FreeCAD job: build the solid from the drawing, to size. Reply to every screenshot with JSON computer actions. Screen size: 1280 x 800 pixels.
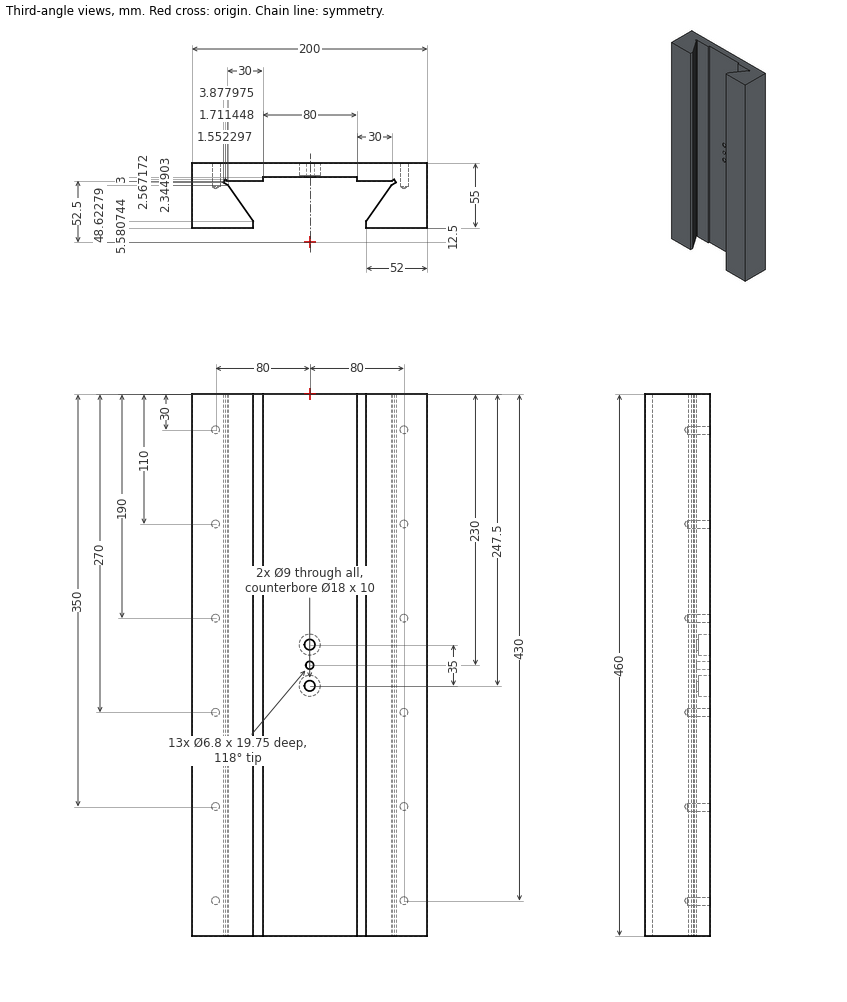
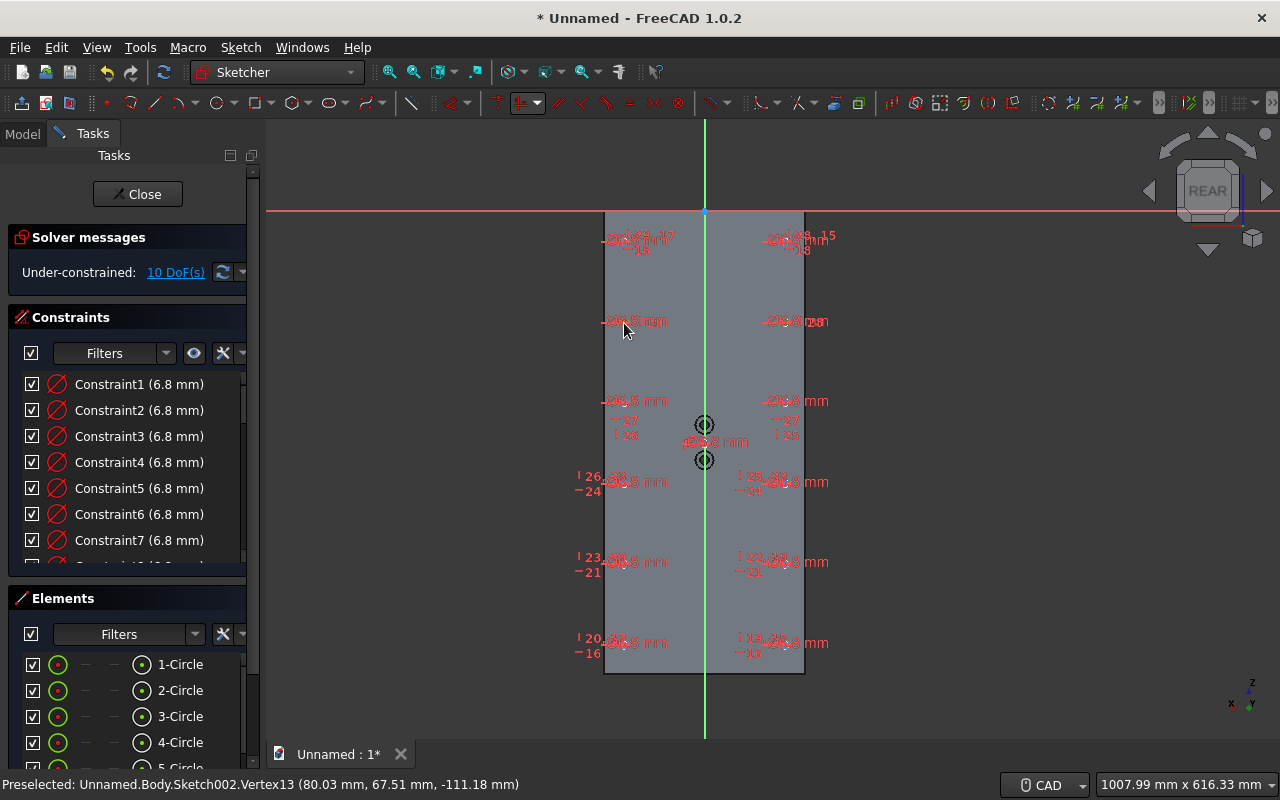
{"action": "key", "text": "h"}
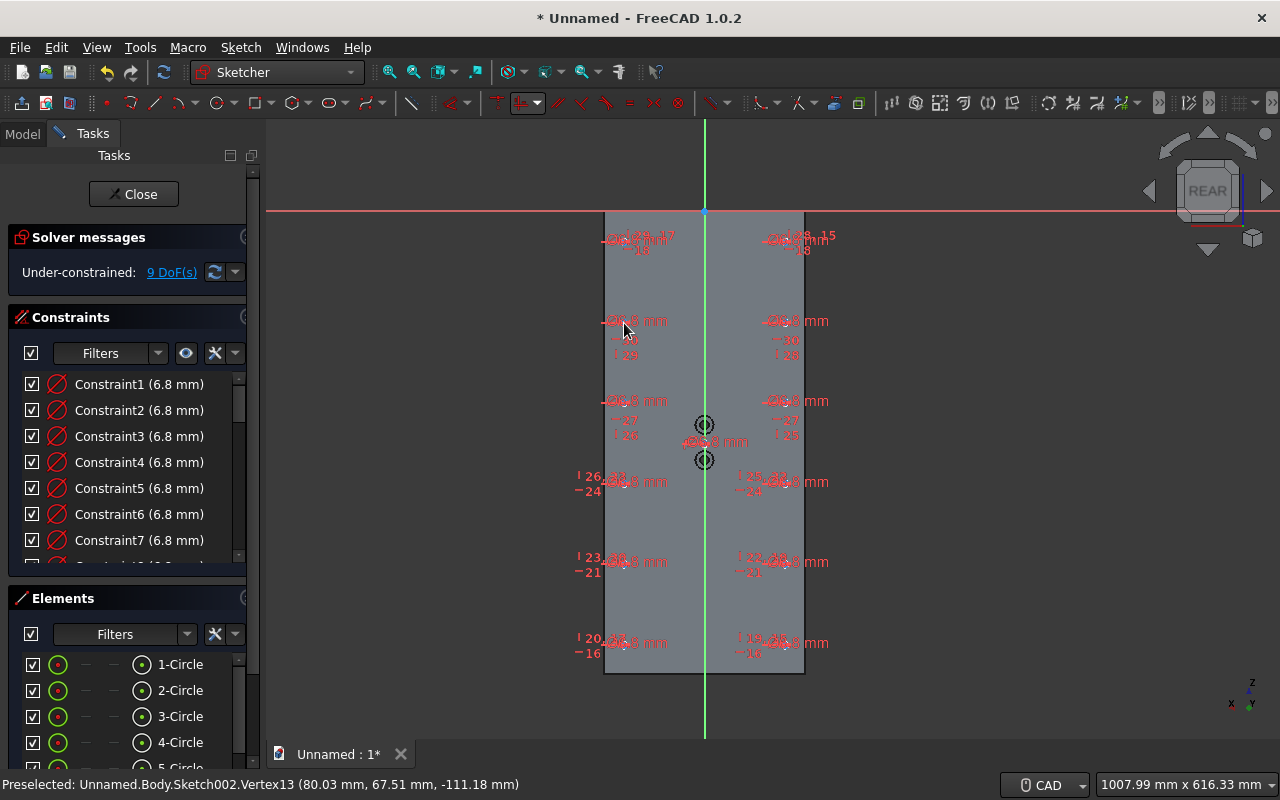
{"action": "left_click", "coordinate": [450, 104]}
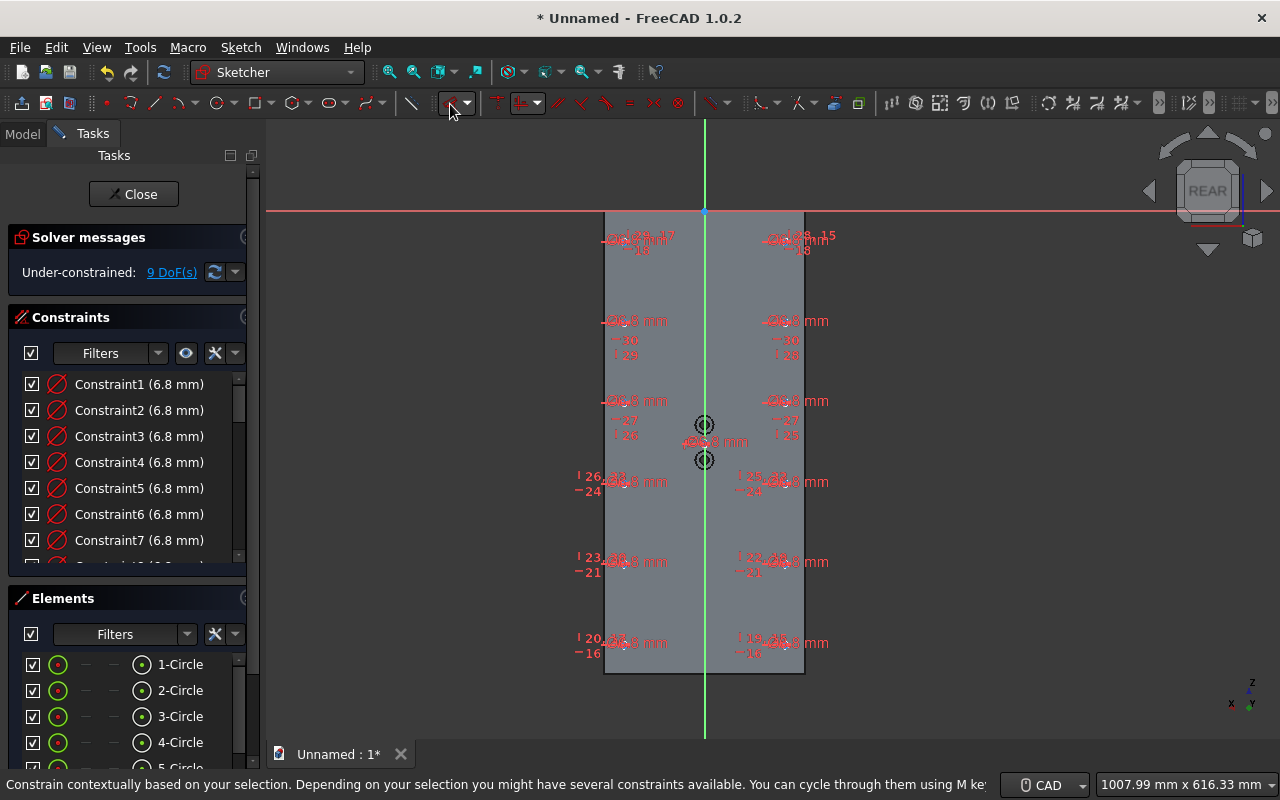
{"action": "left_click", "coordinate": [624, 645]}
{"action": "left_click", "coordinate": [664, 177]}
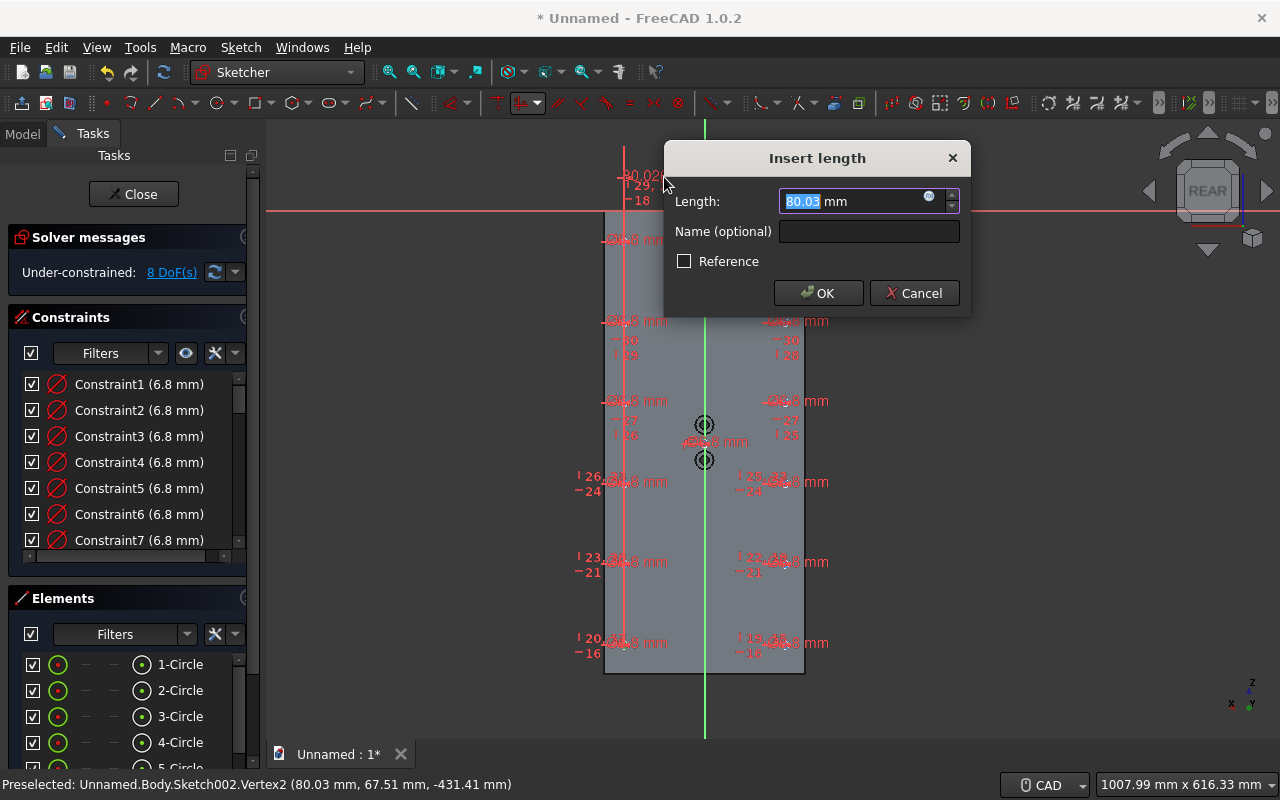
{"action": "type", "text": "80"}
{"action": "key", "text": "Return"}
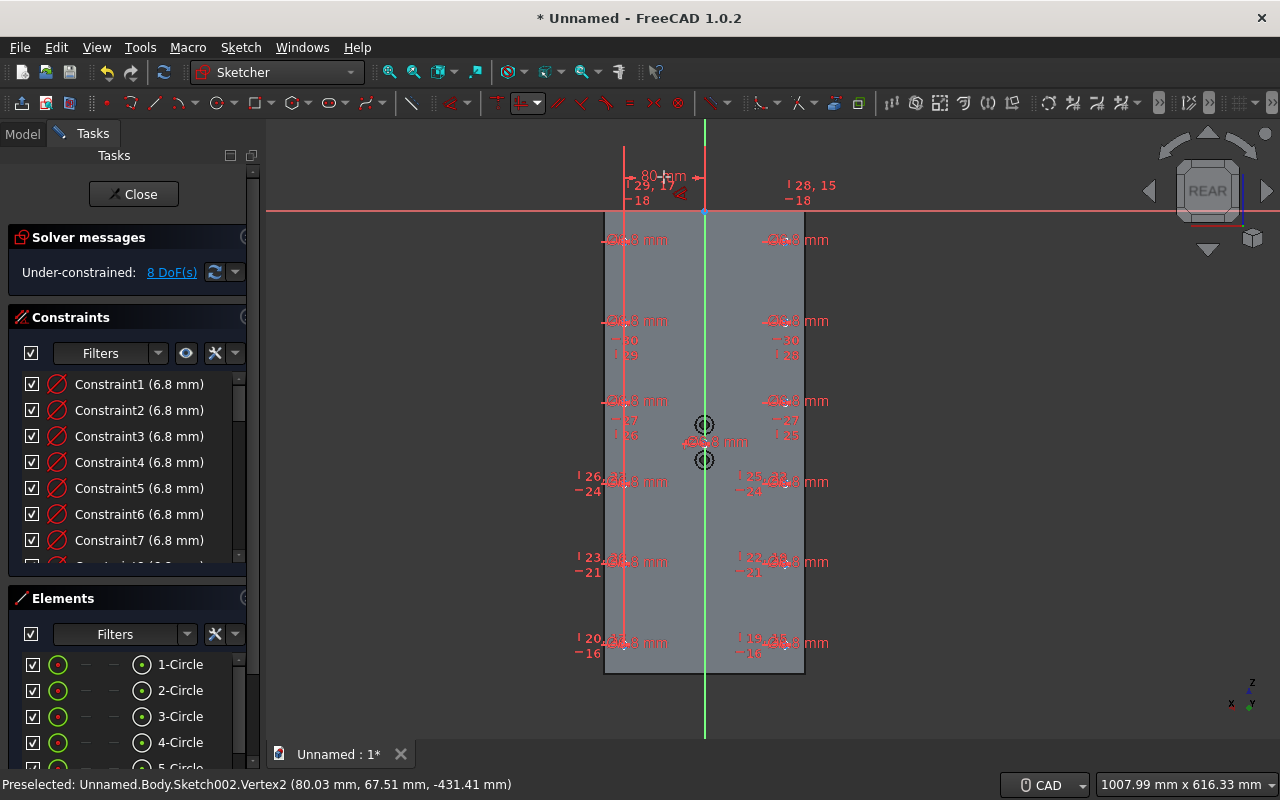
{"action": "left_click", "coordinate": [785, 242]}
{"action": "left_click", "coordinate": [745, 177]}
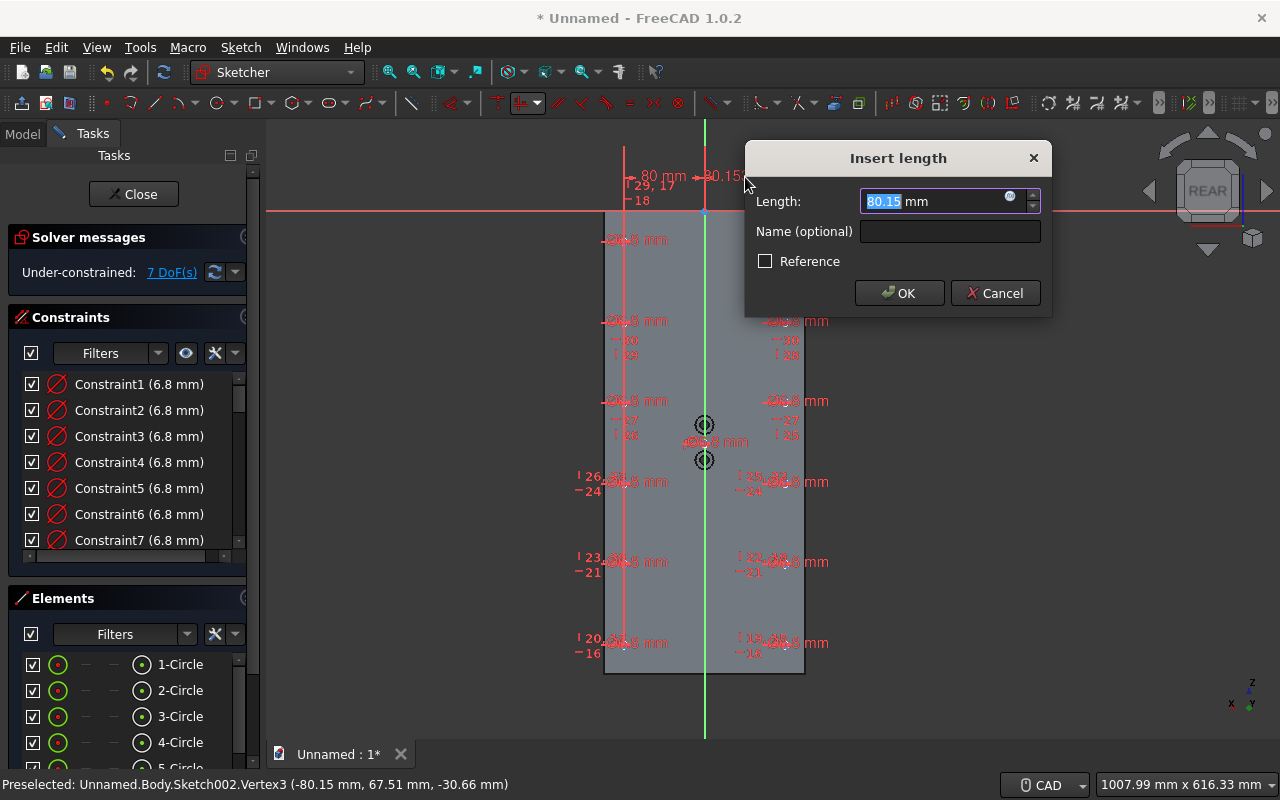
{"action": "type", "text": "80"}
{"action": "key", "text": "Return"}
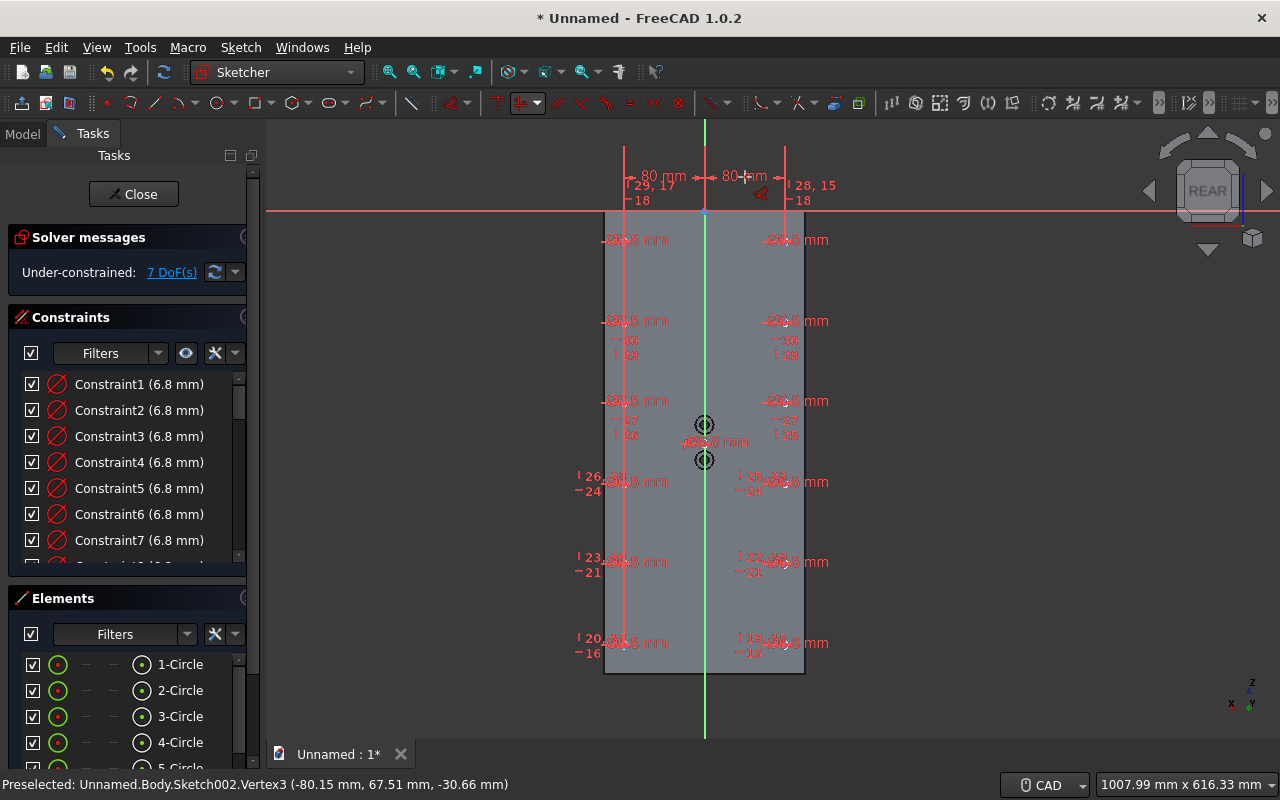
{"action": "scroll", "coordinate": [785, 242], "scroll_direction": "up", "scroll_amount": 2}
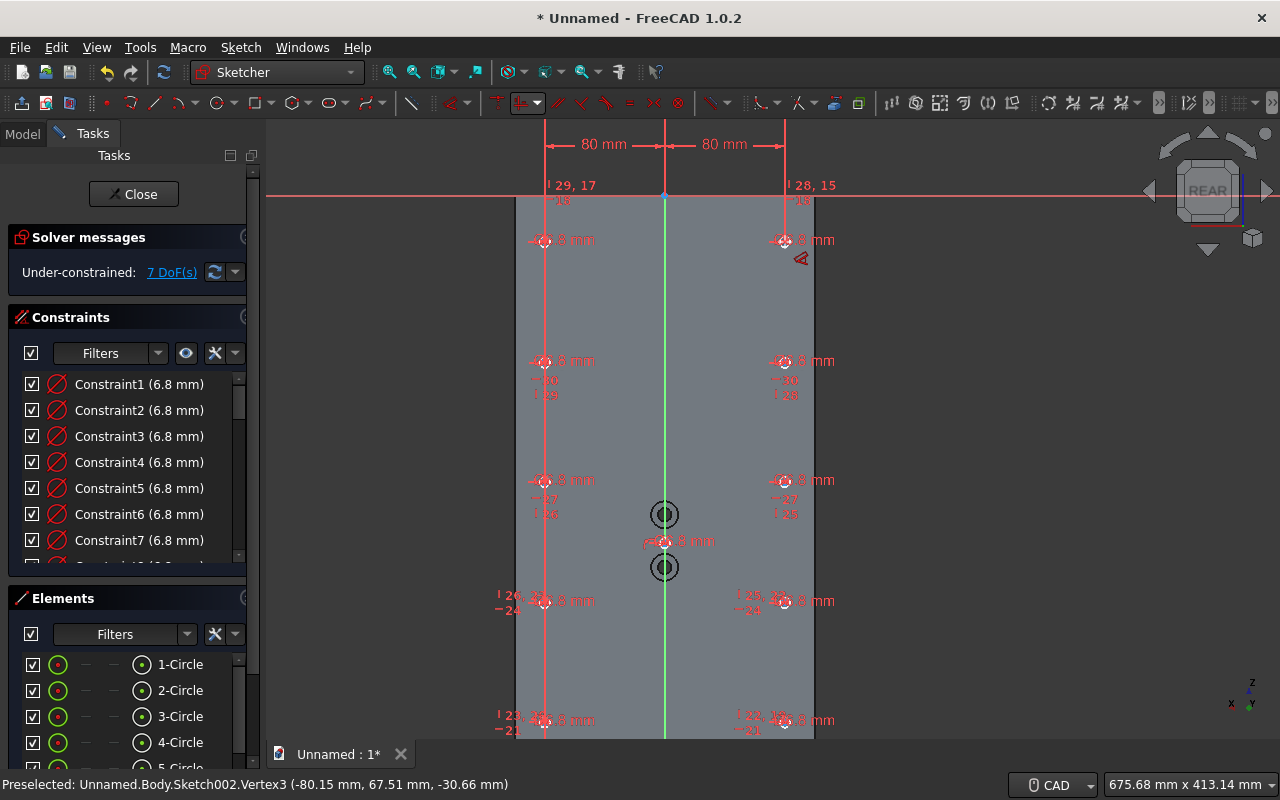
{"action": "left_click", "coordinate": [785, 242]}
{"action": "left_click", "coordinate": [819, 219]}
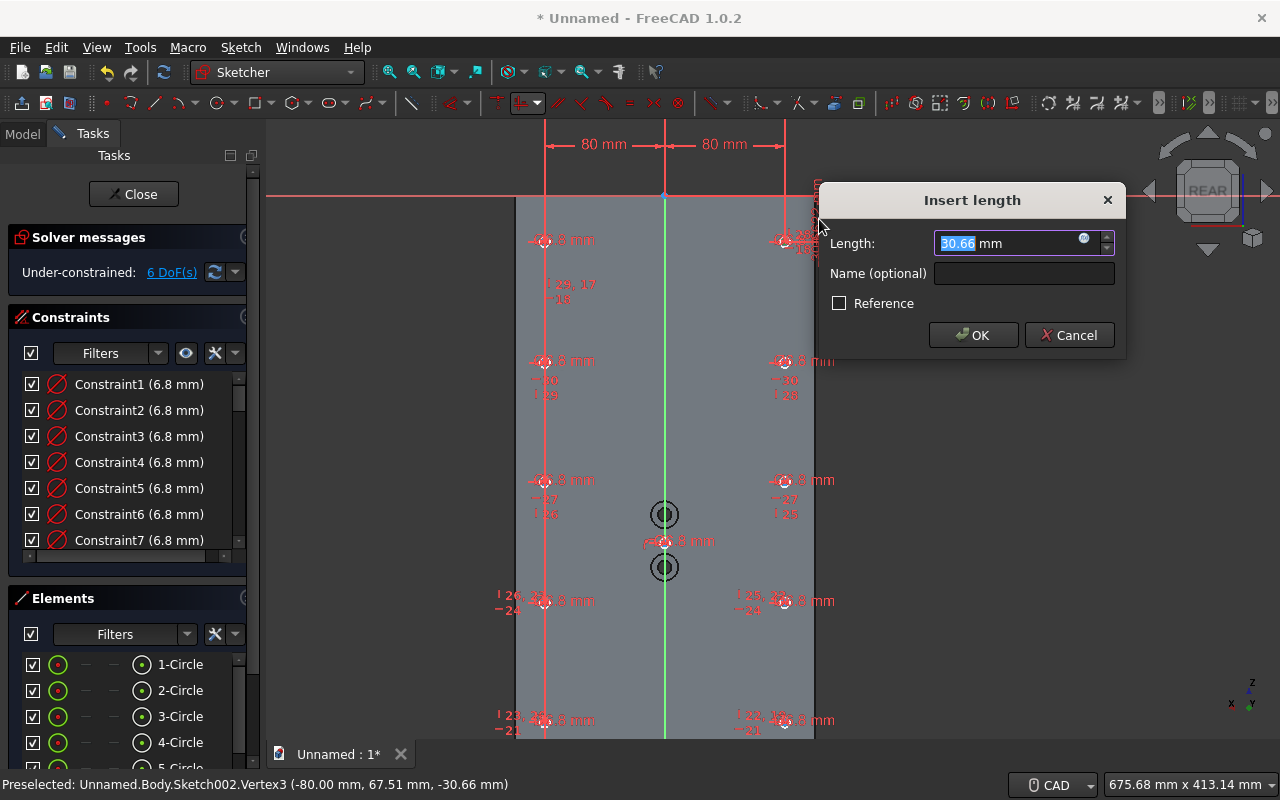
{"action": "type", "text": "30"}
{"action": "key", "text": "Return"}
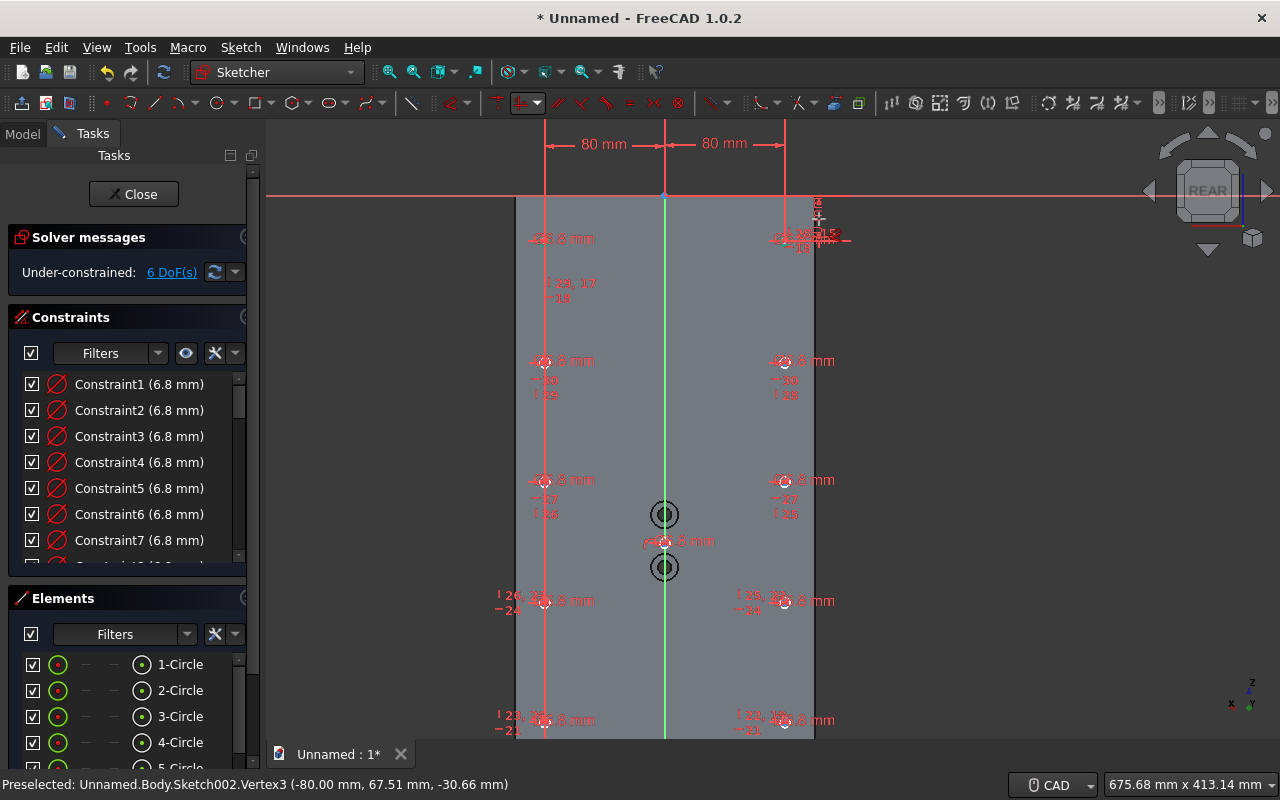
{"action": "left_click", "coordinate": [665, 543]}
{"action": "left_click", "coordinate": [699, 370]}